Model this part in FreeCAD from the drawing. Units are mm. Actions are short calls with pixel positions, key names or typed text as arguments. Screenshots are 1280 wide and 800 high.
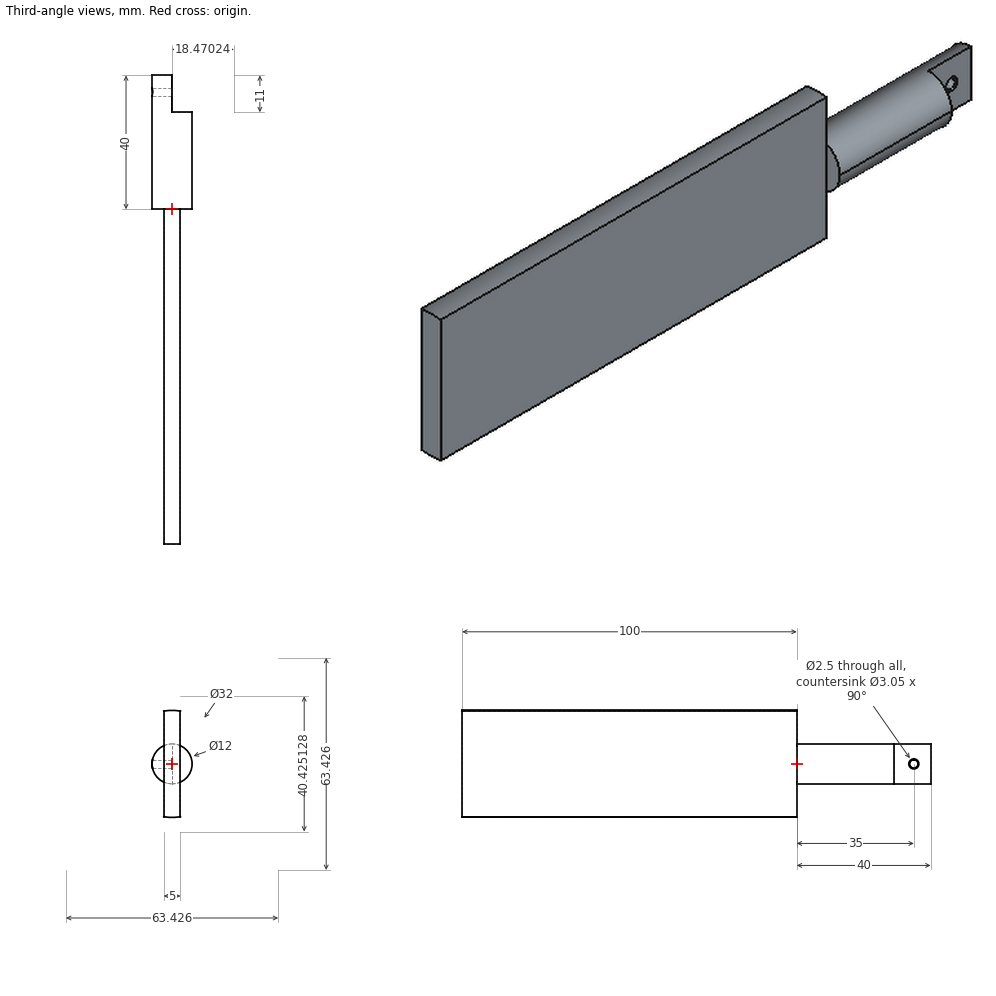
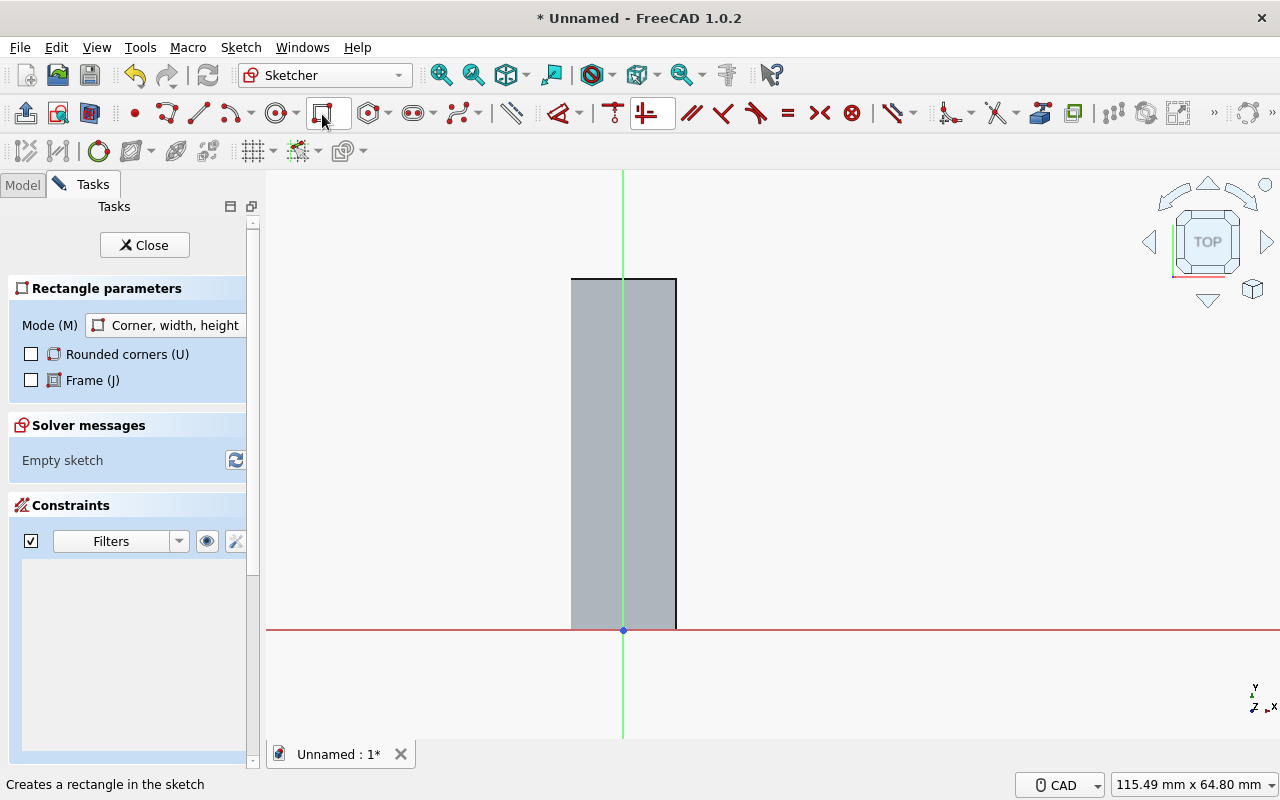
click(623, 279)
move(786, 375)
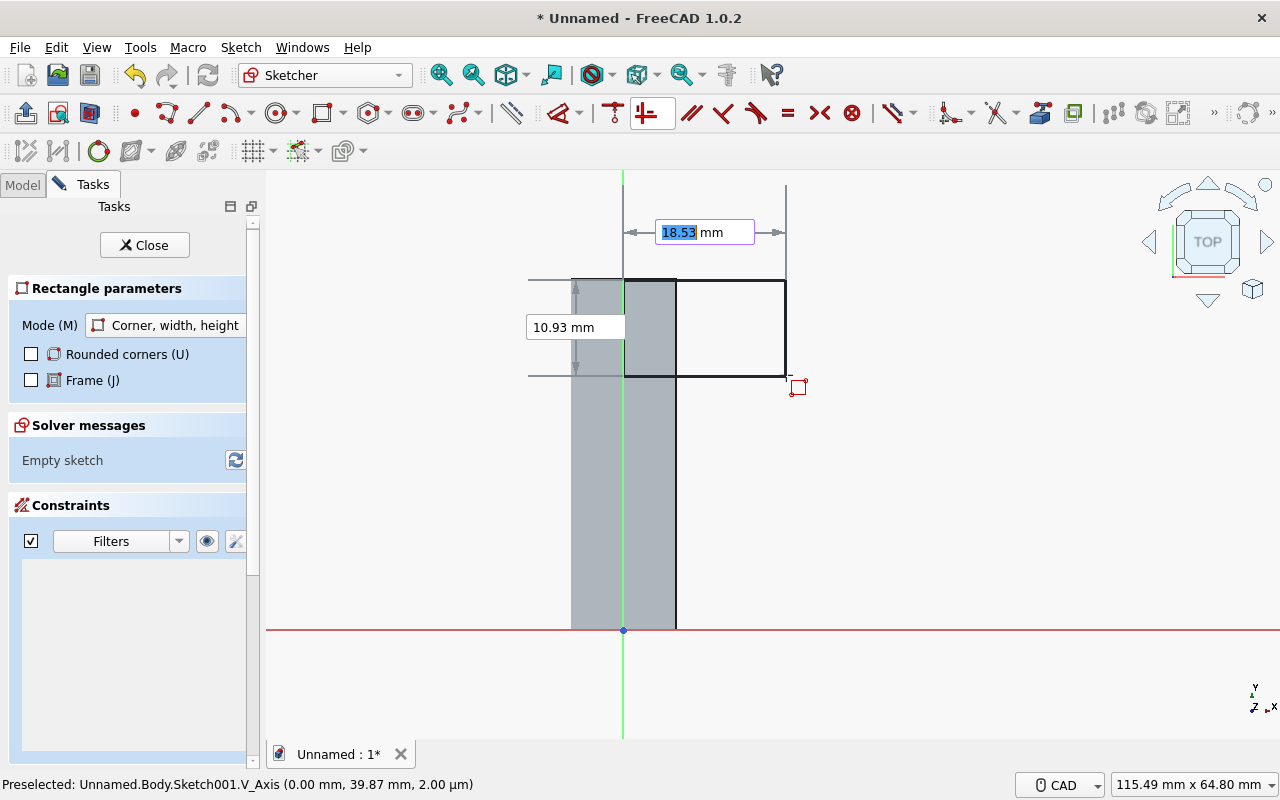
text(18.47024)
key(Tab)
text(11)
key(Return)
key(Escape)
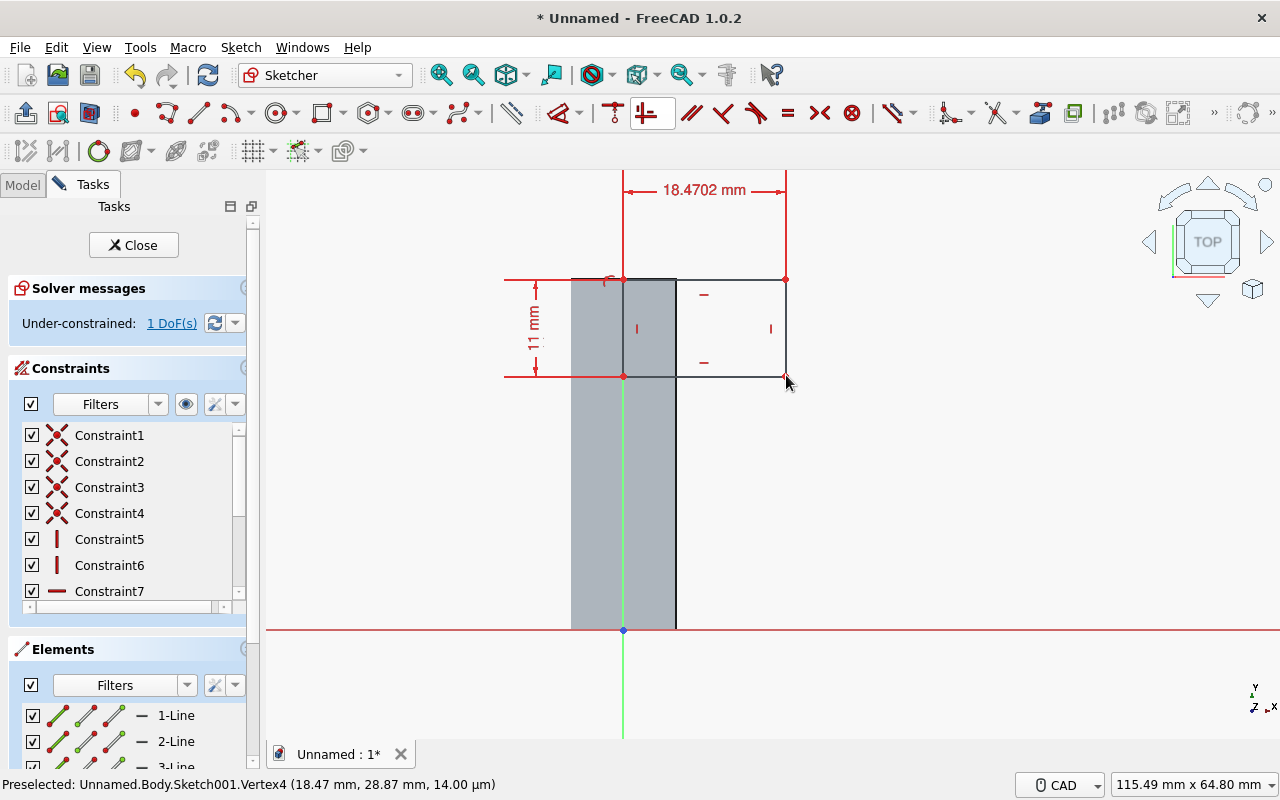
click(623, 280)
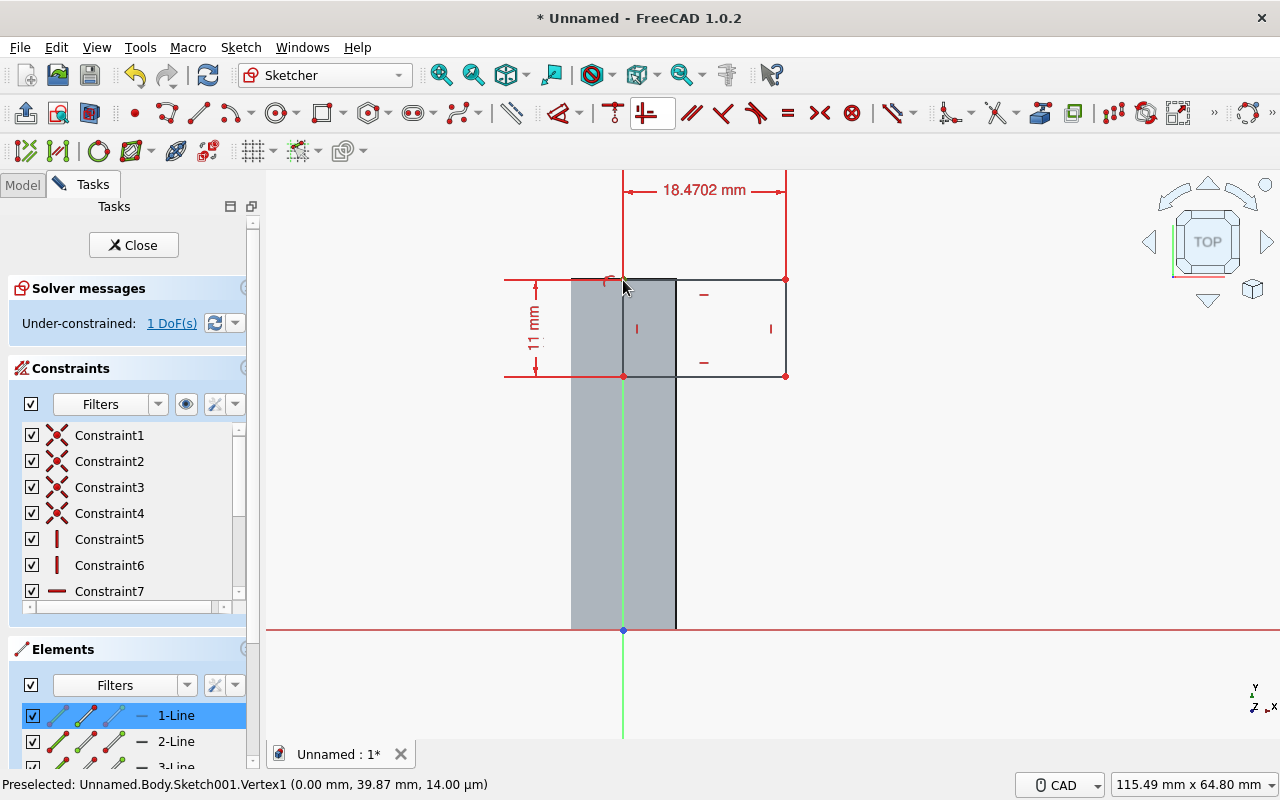
key(i)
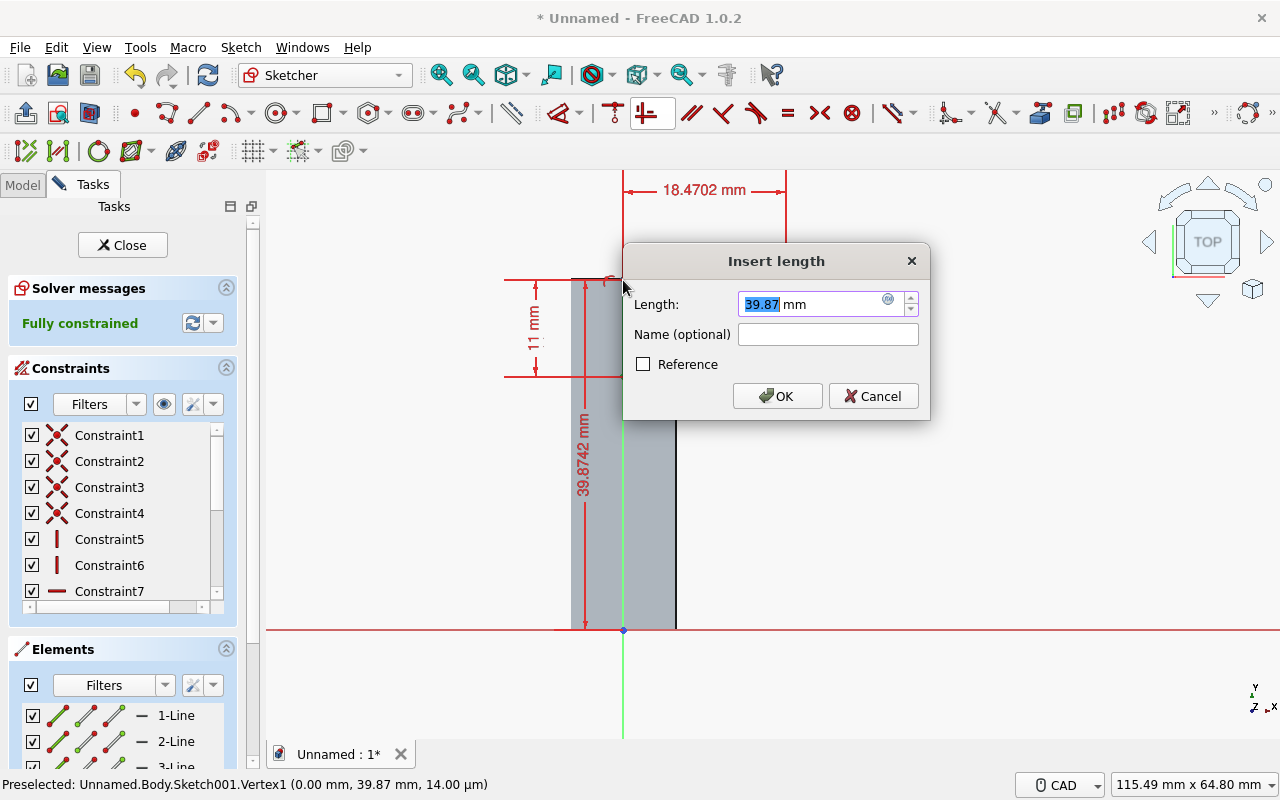
text(40)
key(Return)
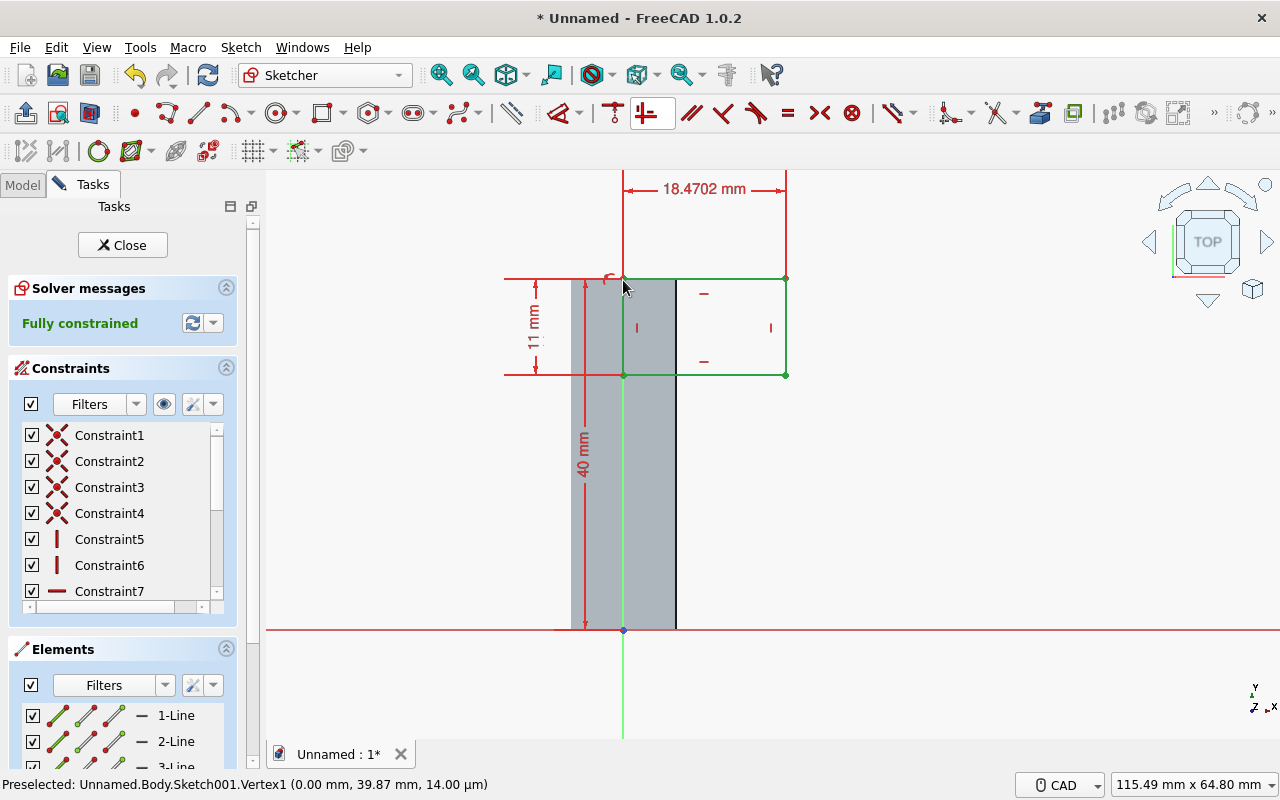
click(123, 245)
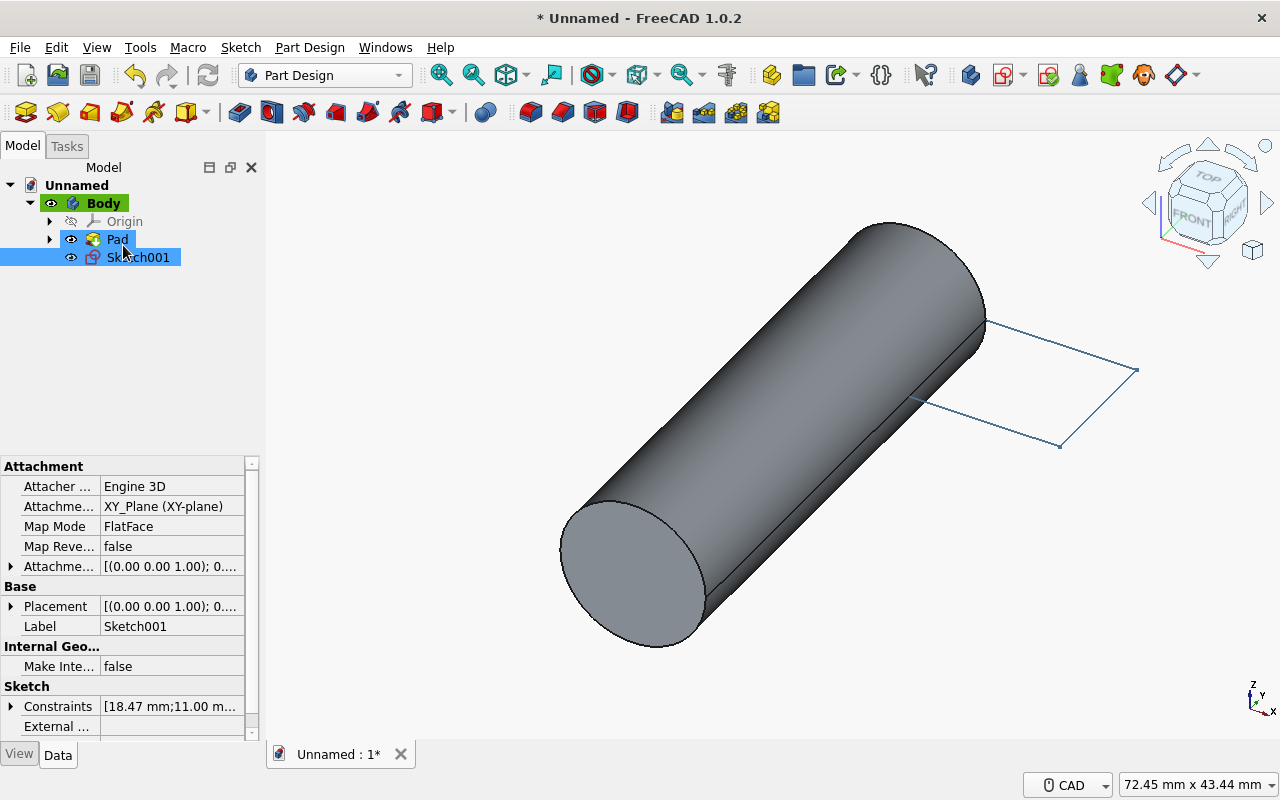
click(240, 112)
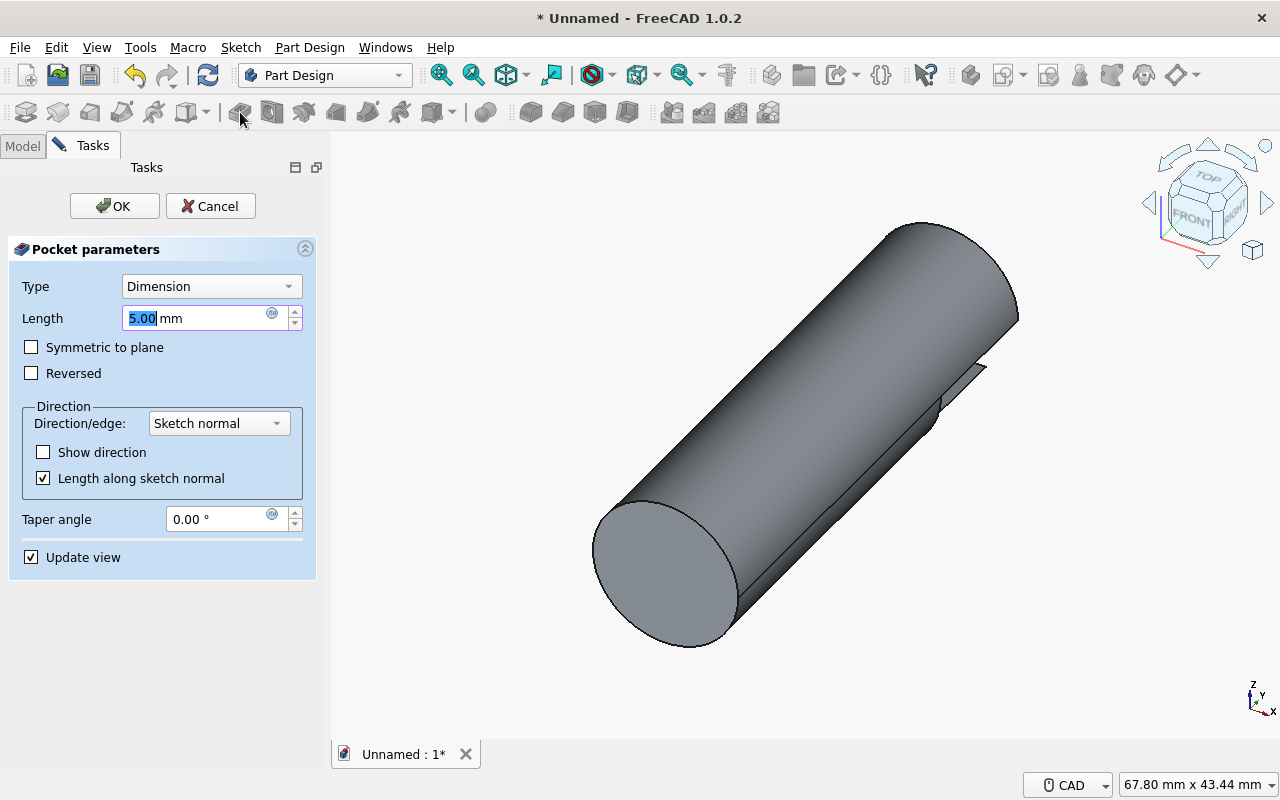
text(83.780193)
key(Tab)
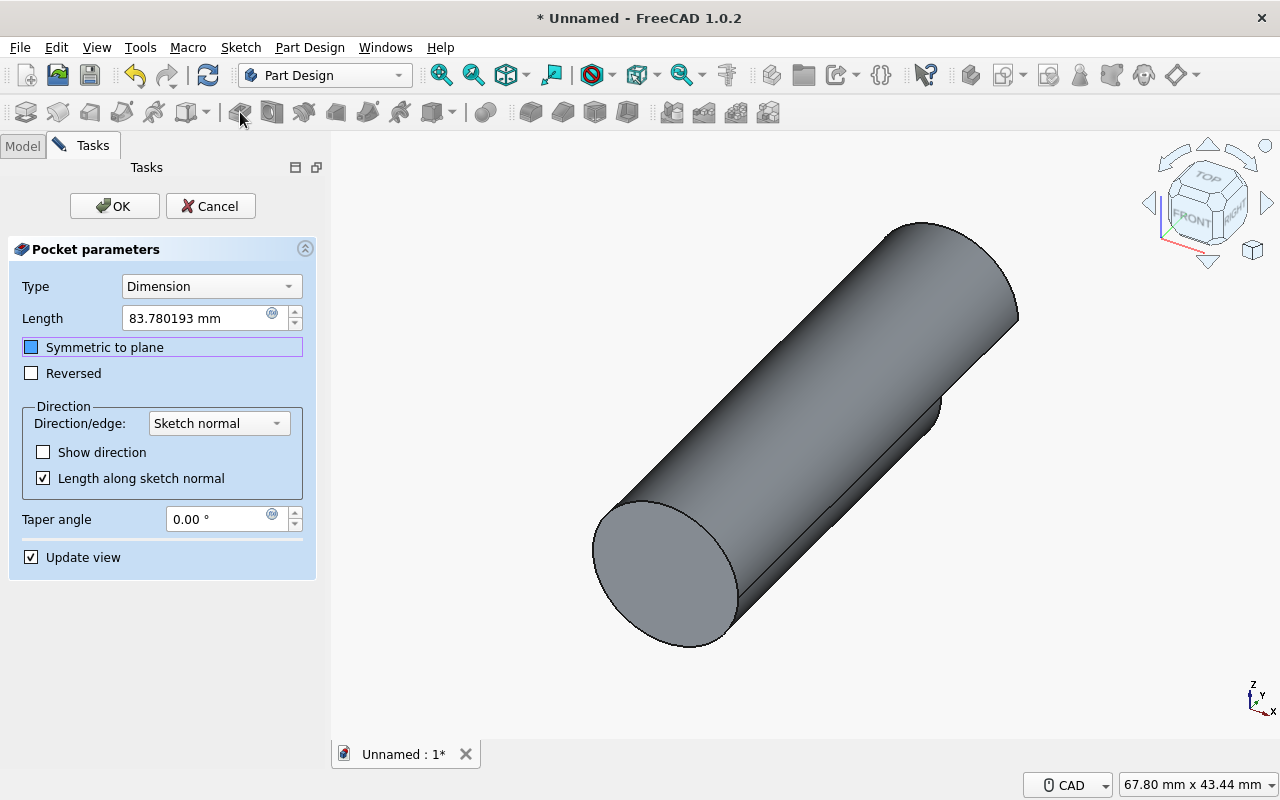
click(30, 347)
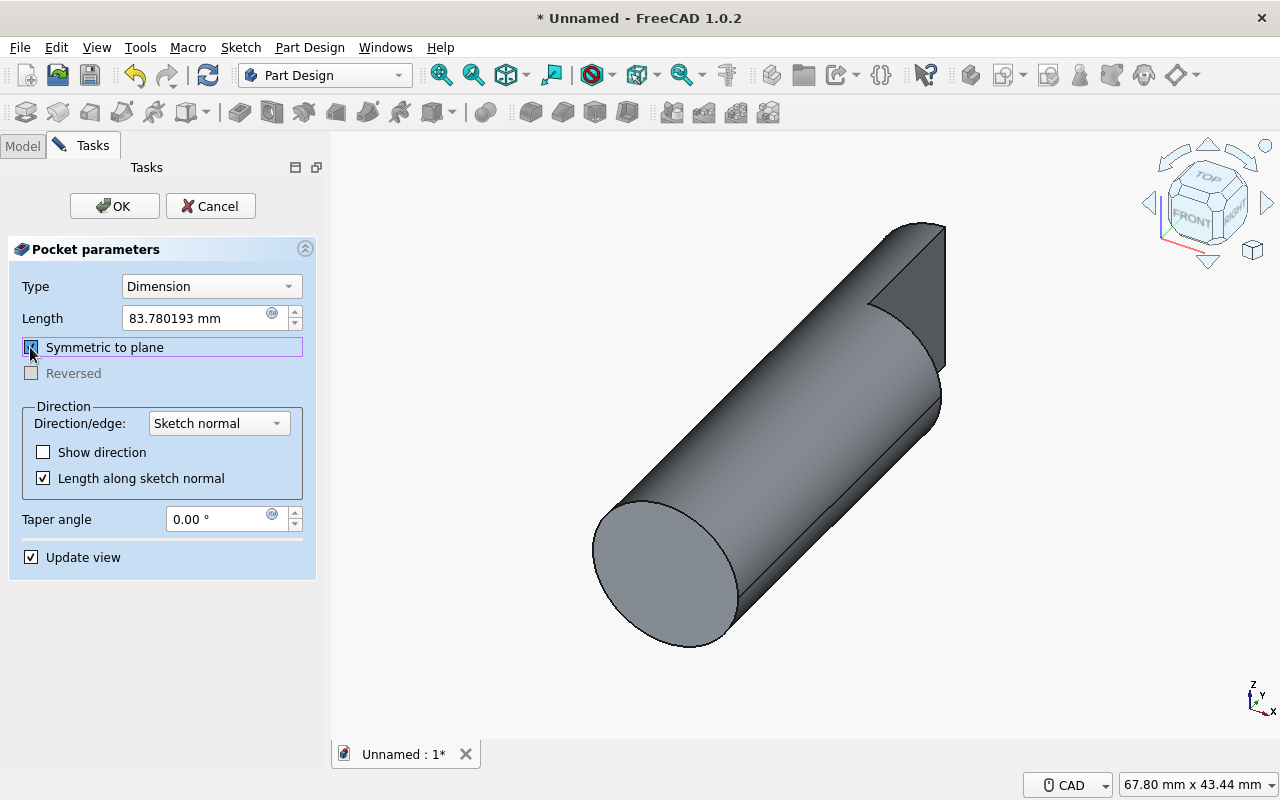
click(115, 206)